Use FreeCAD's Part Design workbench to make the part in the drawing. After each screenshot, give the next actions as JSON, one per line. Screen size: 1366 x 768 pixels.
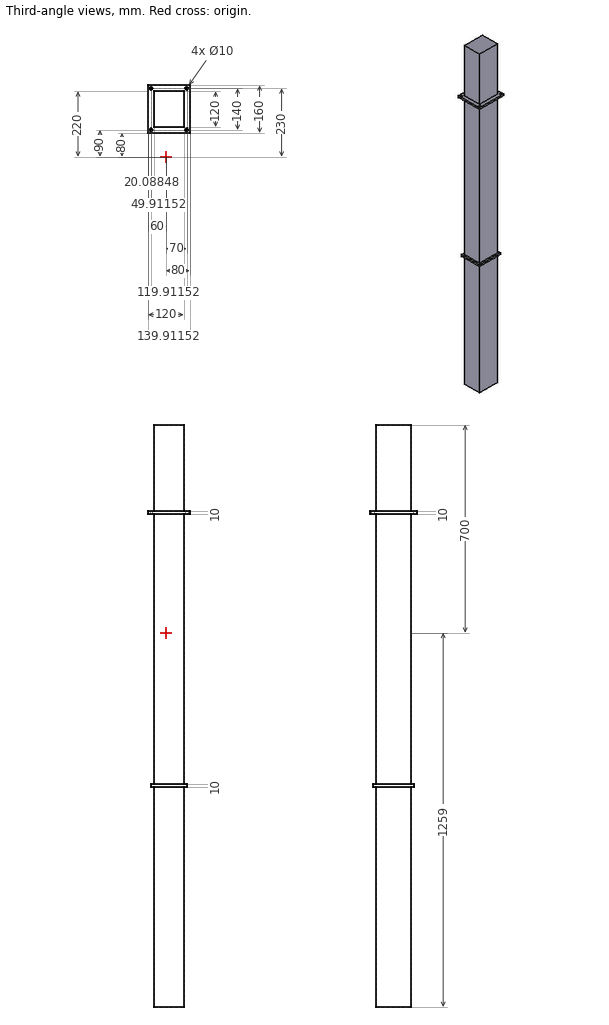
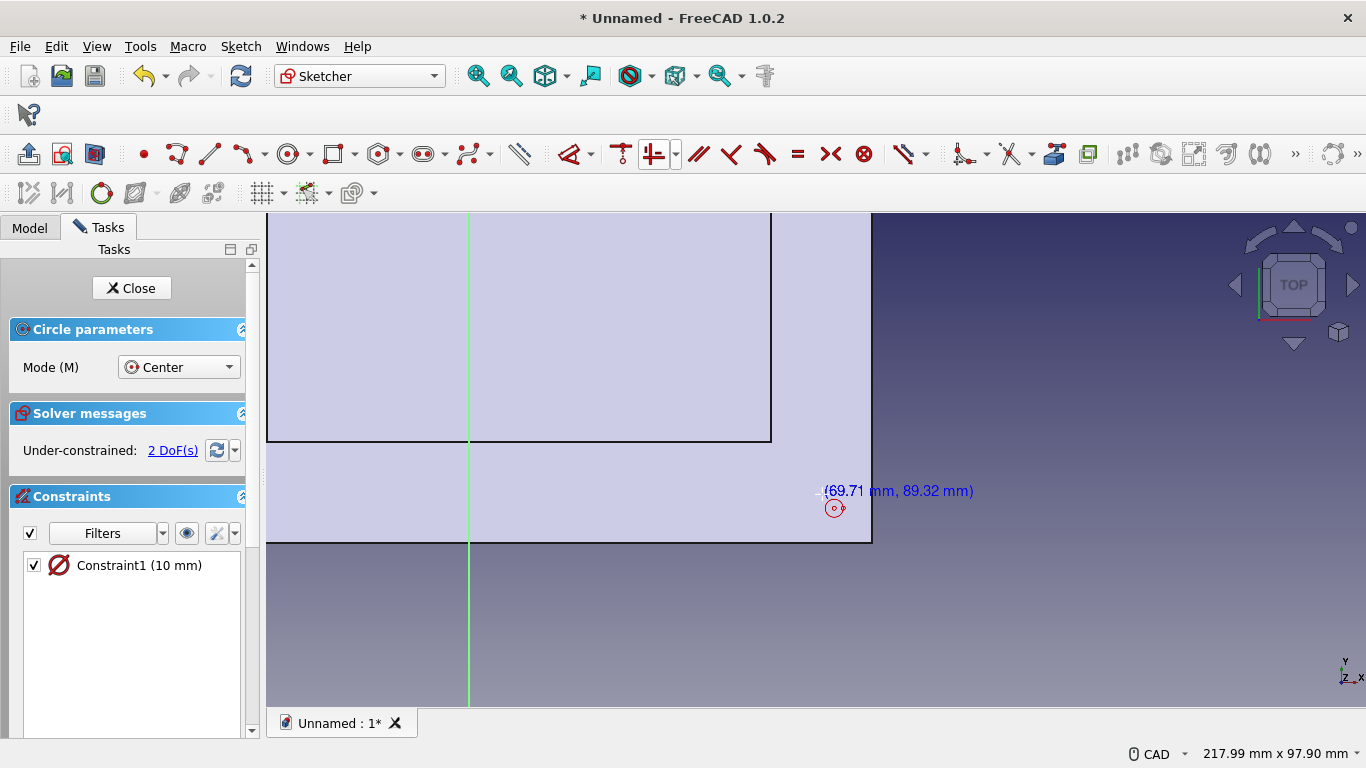
{"action": "scroll", "coordinate": [822, 495], "scroll_direction": "down", "scroll_amount": 7}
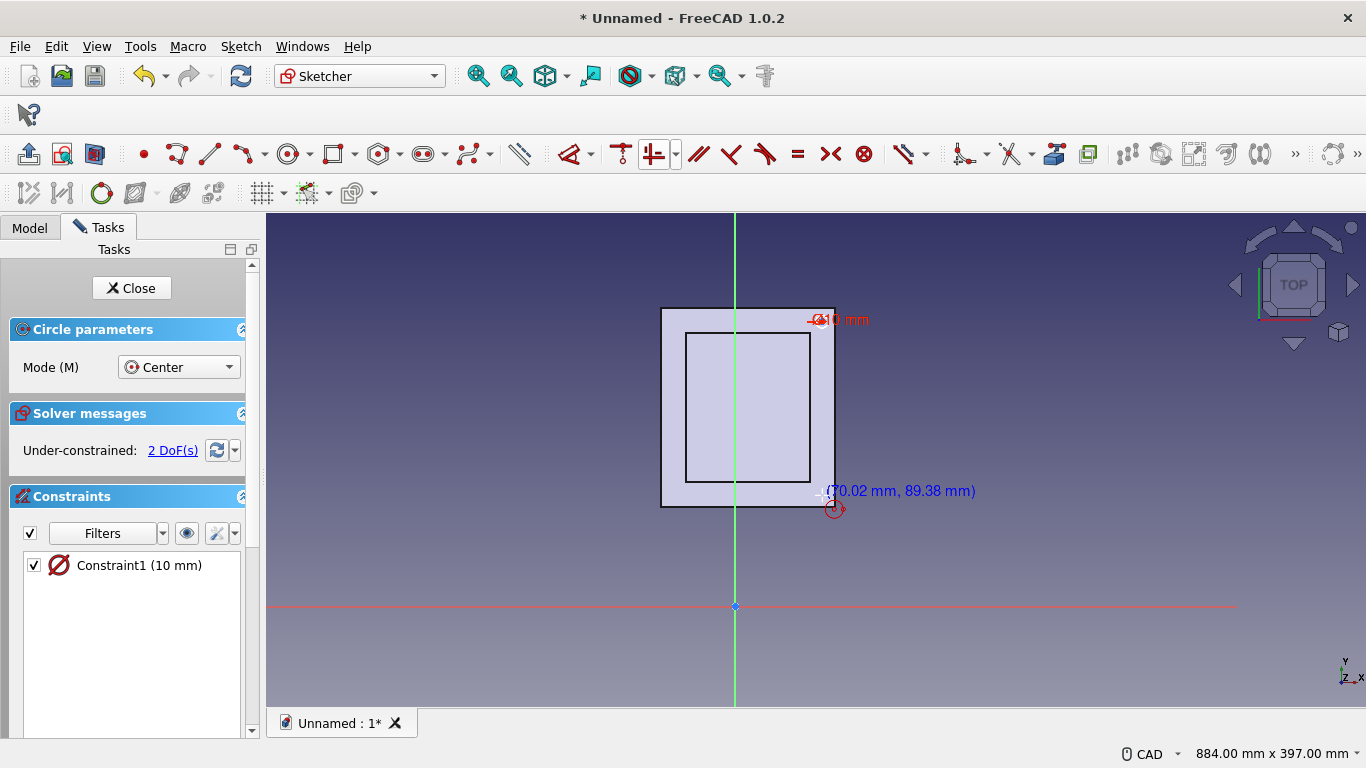
{"action": "left_click", "coordinate": [822, 495]}
{"action": "mouse_move", "coordinate": [827, 491]}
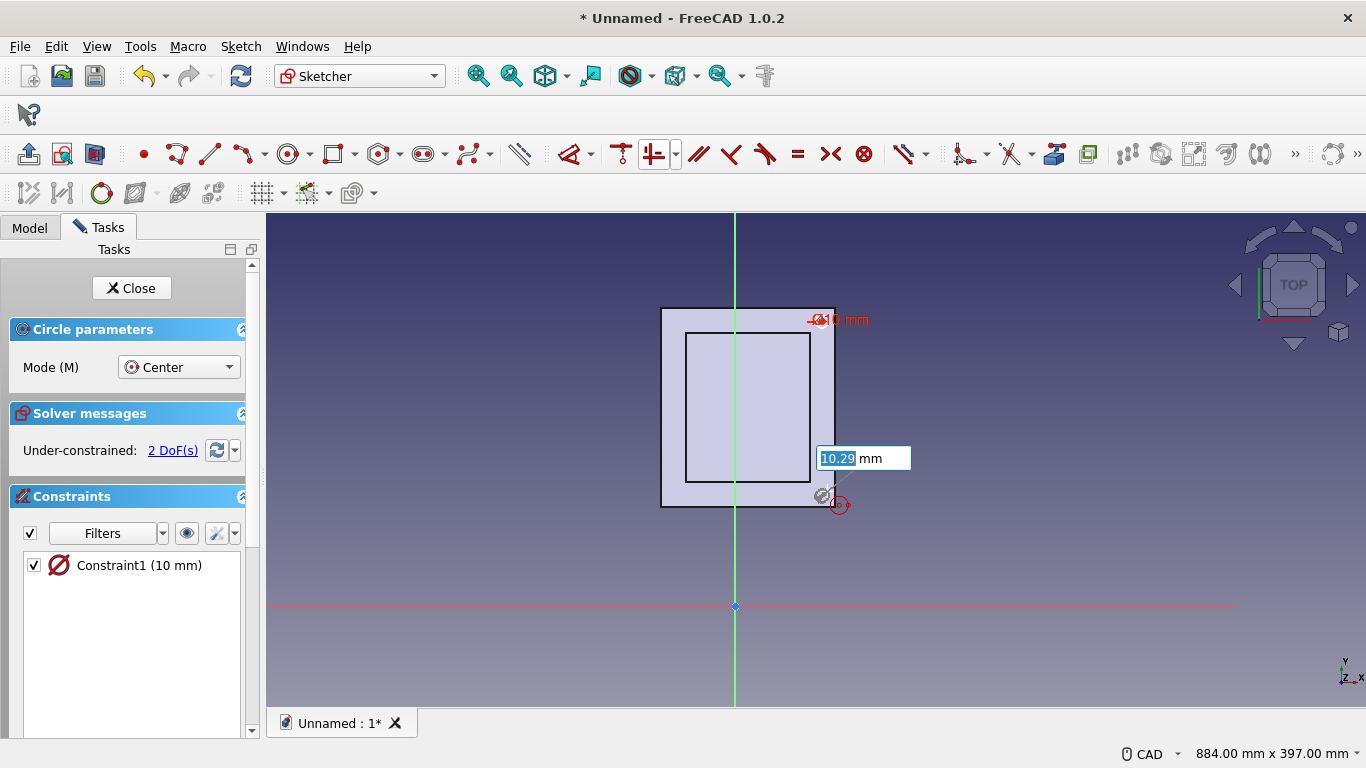
{"action": "type", "text": "10"}
{"action": "key", "text": "Return"}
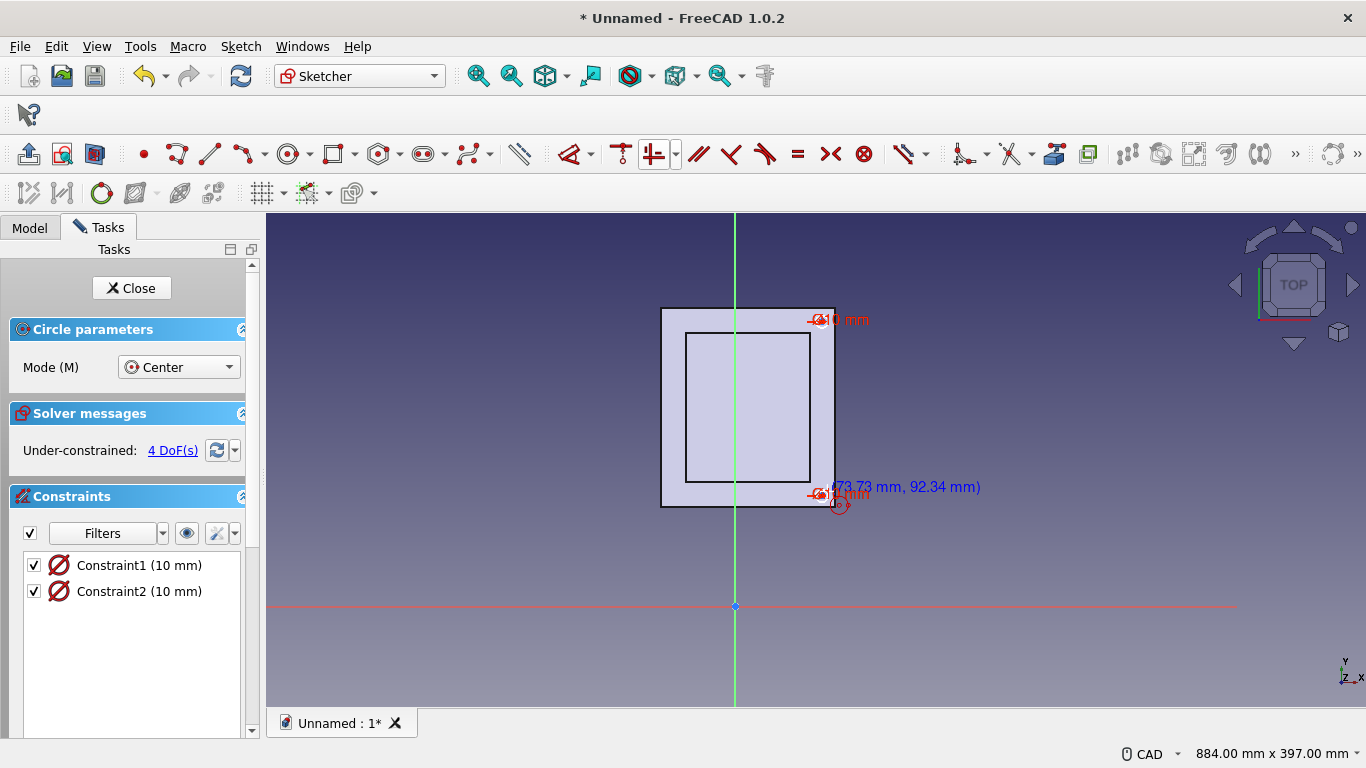
{"action": "scroll", "coordinate": [673, 495], "scroll_direction": "up", "scroll_amount": 7}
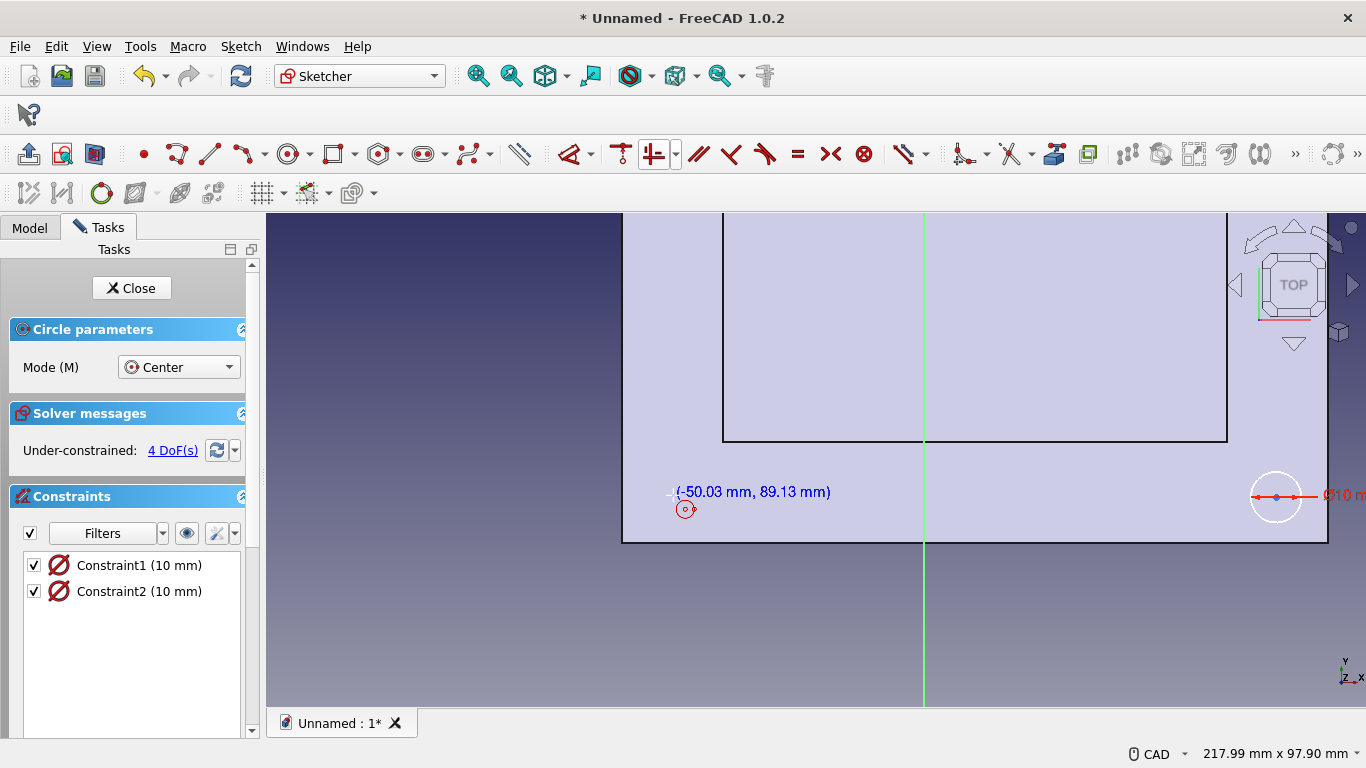
{"action": "scroll", "coordinate": [673, 495], "scroll_direction": "down", "scroll_amount": 7}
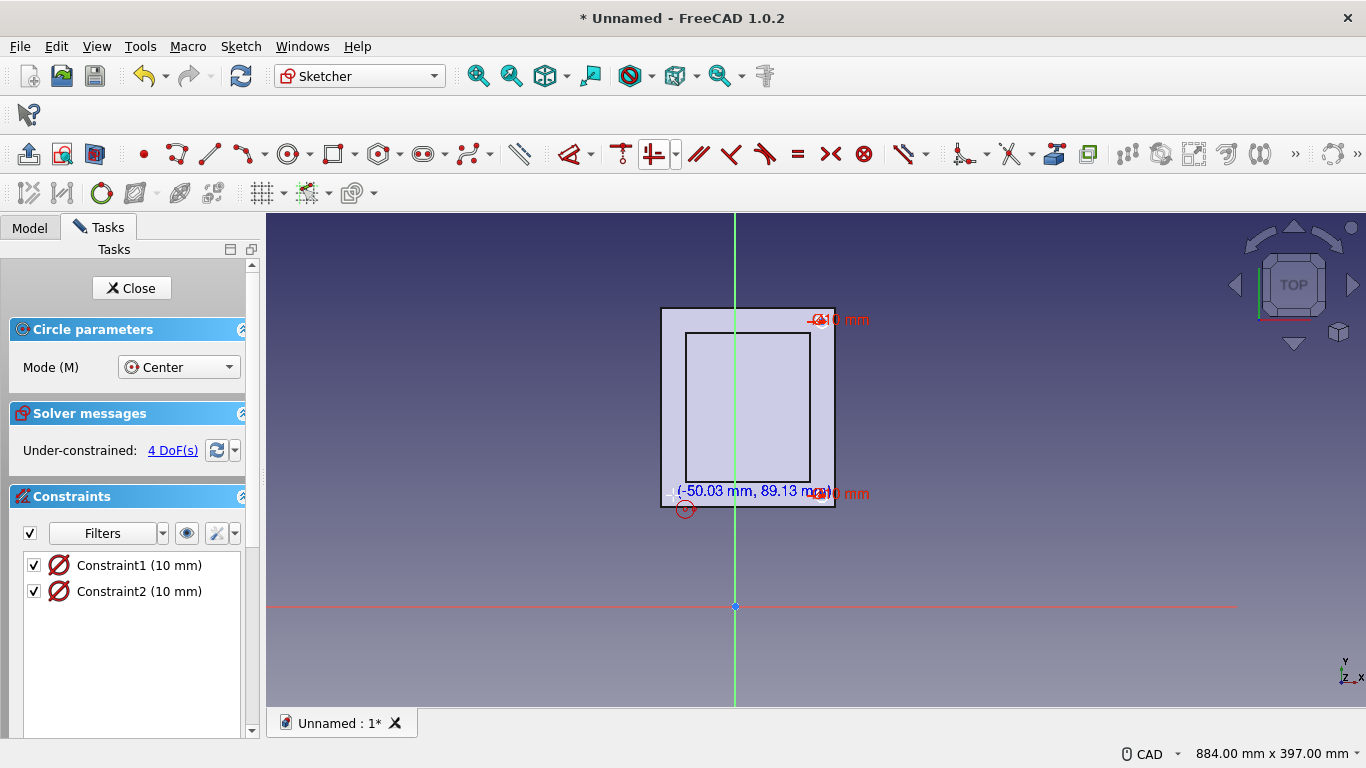
{"action": "left_click", "coordinate": [673, 495]}
{"action": "mouse_move", "coordinate": [678, 491]}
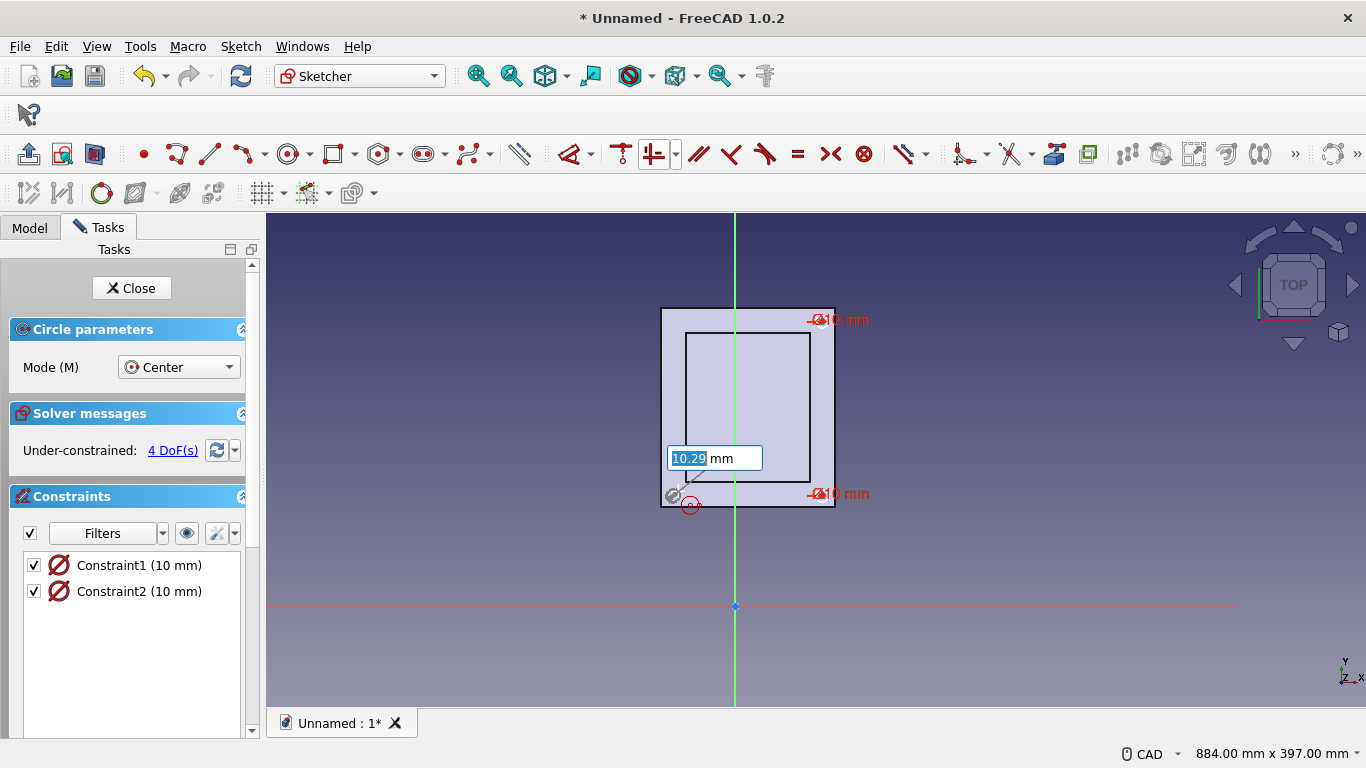
{"action": "type", "text": "10"}
{"action": "key", "text": "Return"}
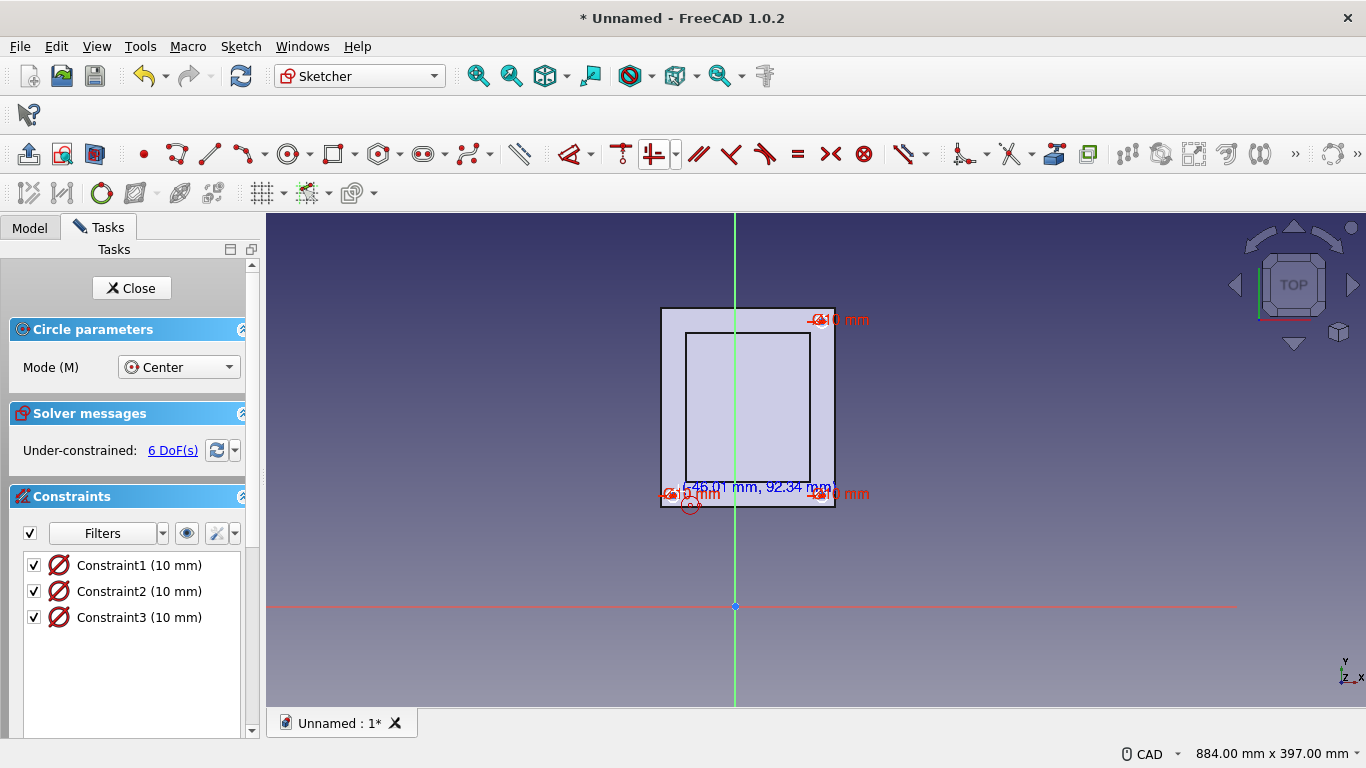
{"action": "scroll", "coordinate": [673, 321], "scroll_direction": "up", "scroll_amount": 7}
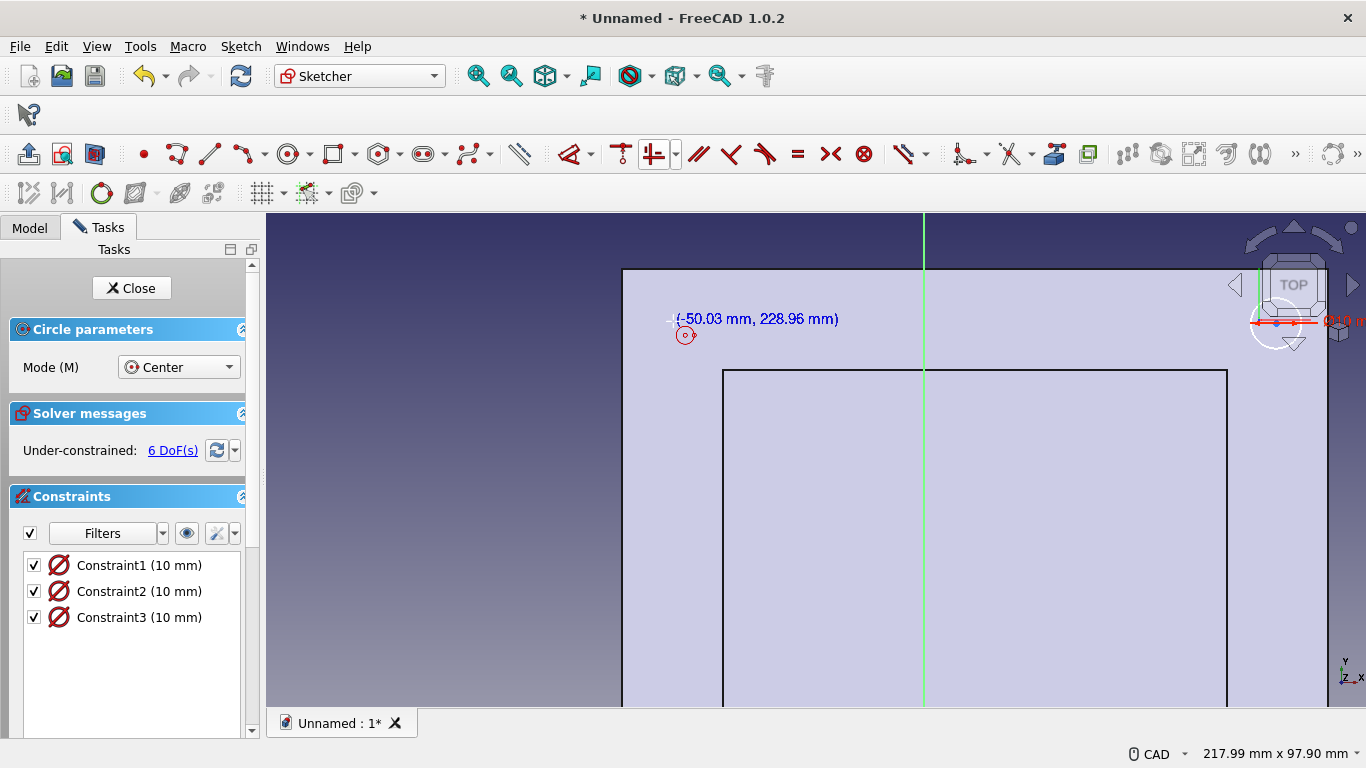
{"action": "scroll", "coordinate": [673, 320], "scroll_direction": "down", "scroll_amount": 7}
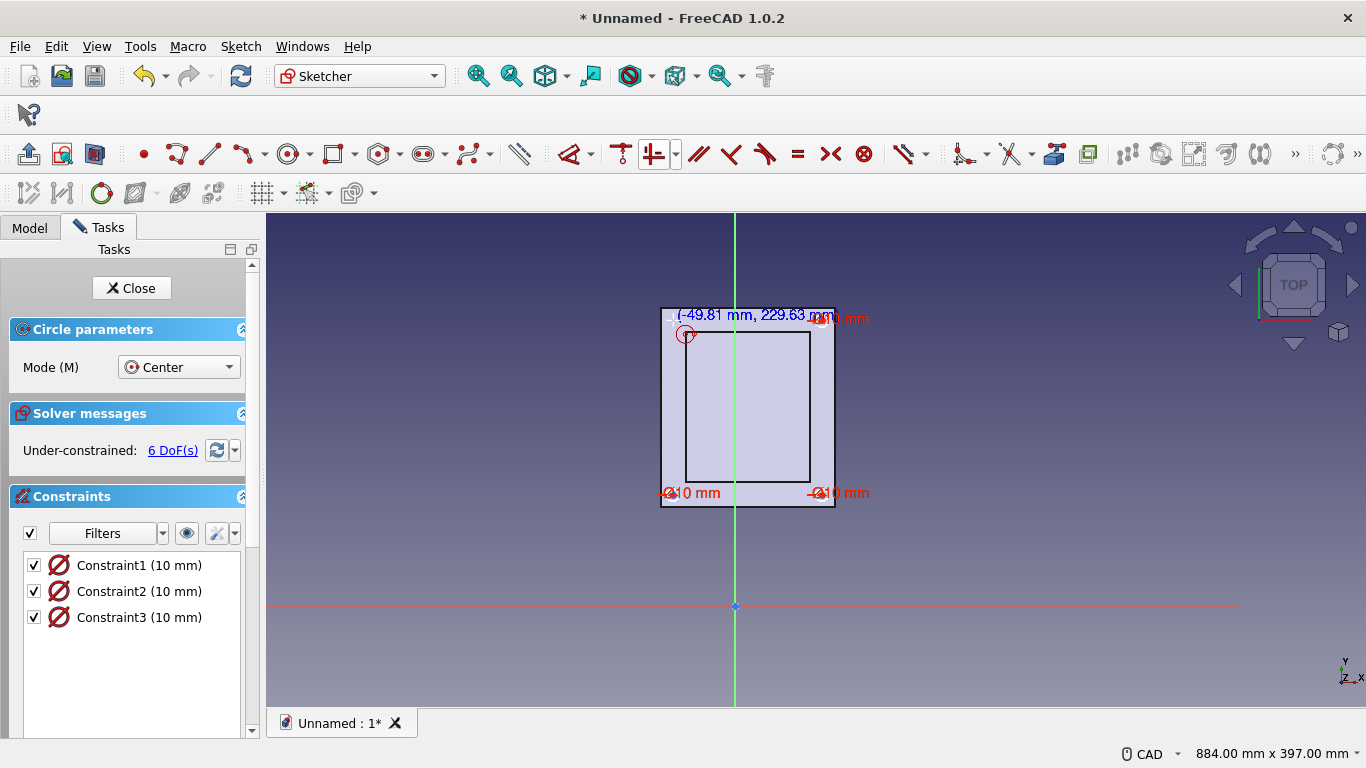
{"action": "left_click", "coordinate": [673, 320]}
{"action": "mouse_move", "coordinate": [678, 316]}